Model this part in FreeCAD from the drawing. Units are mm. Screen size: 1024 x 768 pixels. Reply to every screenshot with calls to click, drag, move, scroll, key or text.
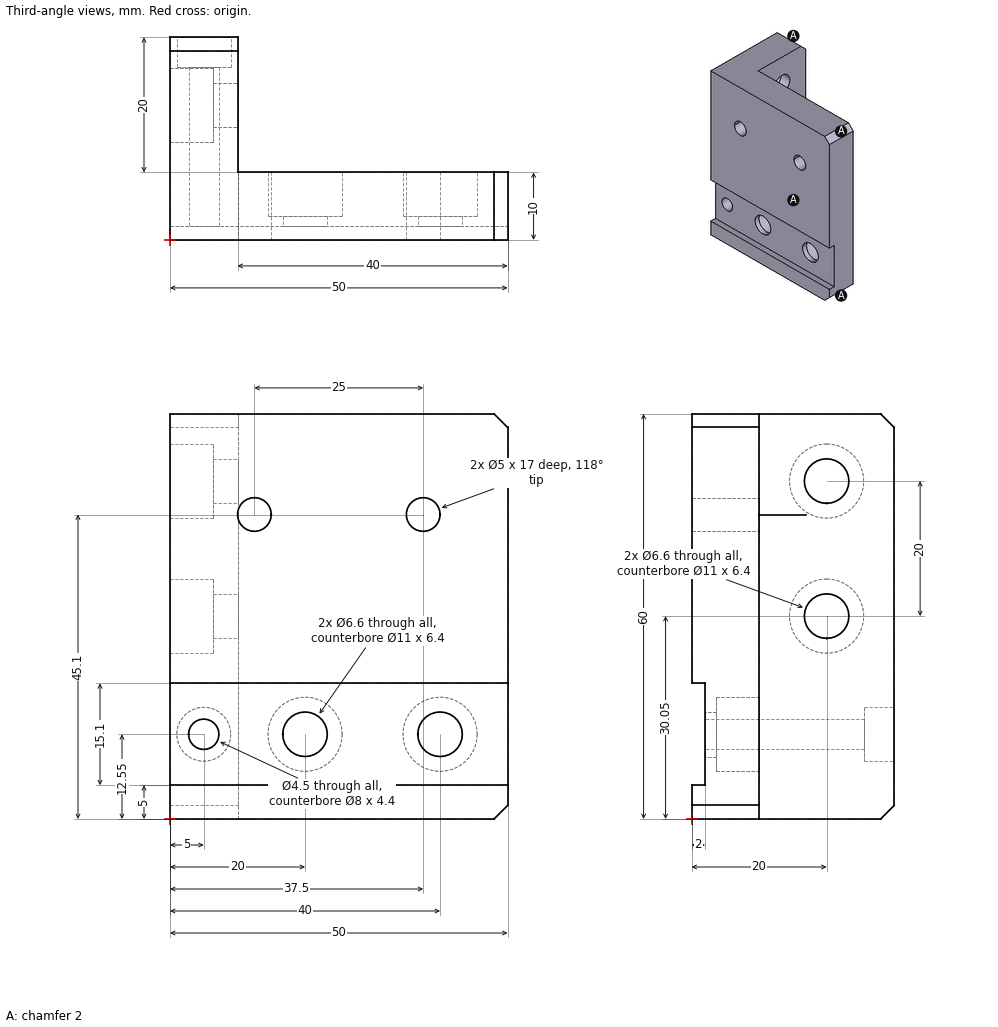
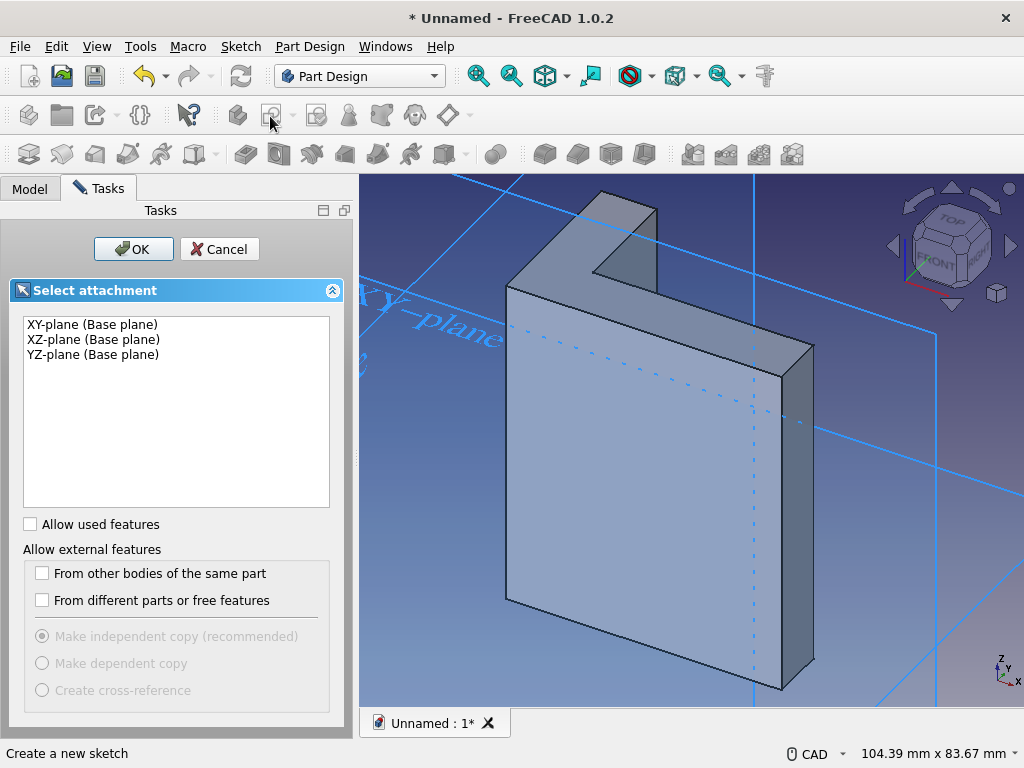
click(84, 340)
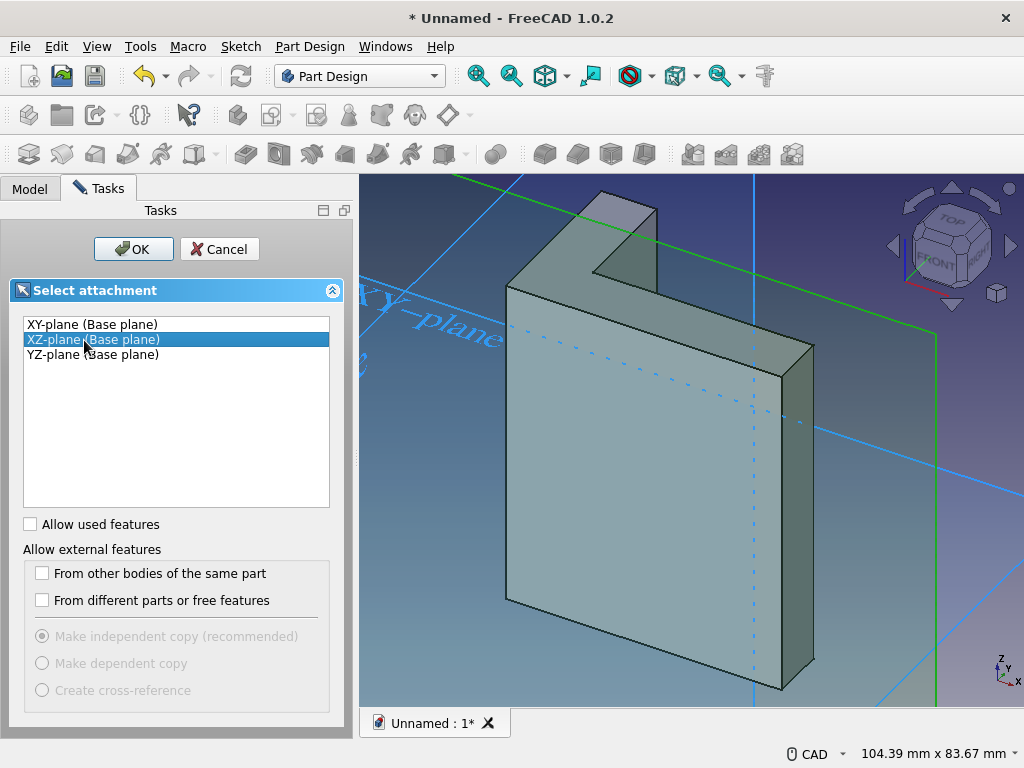
click(134, 249)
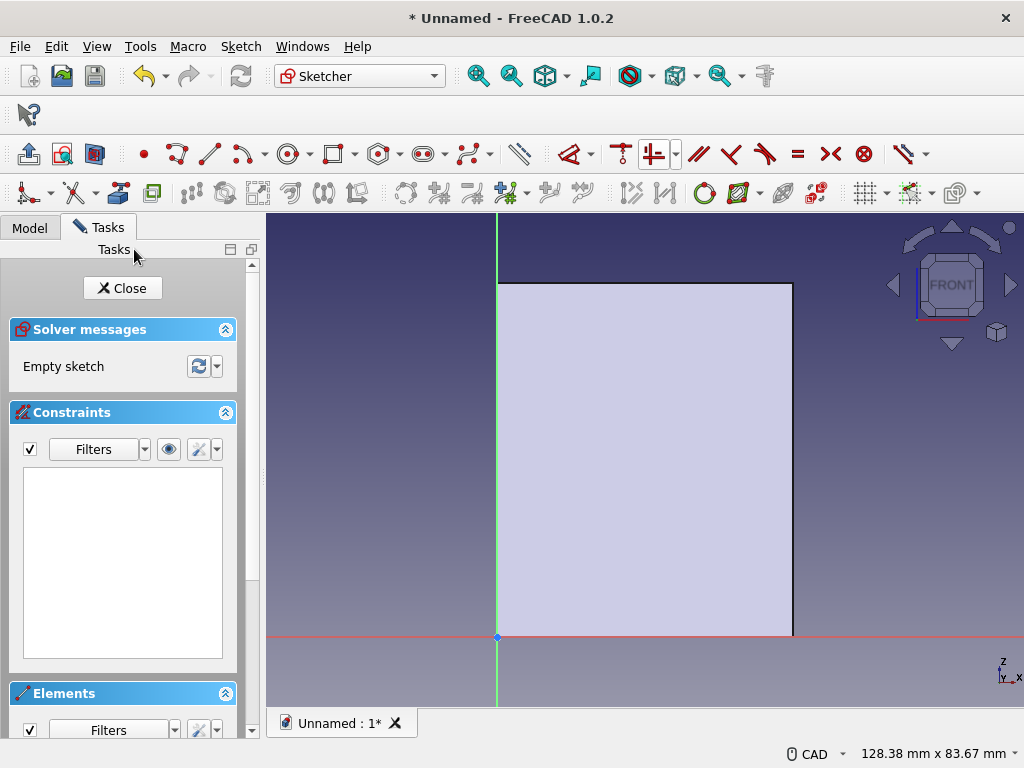
scroll(784, 679, up, 2)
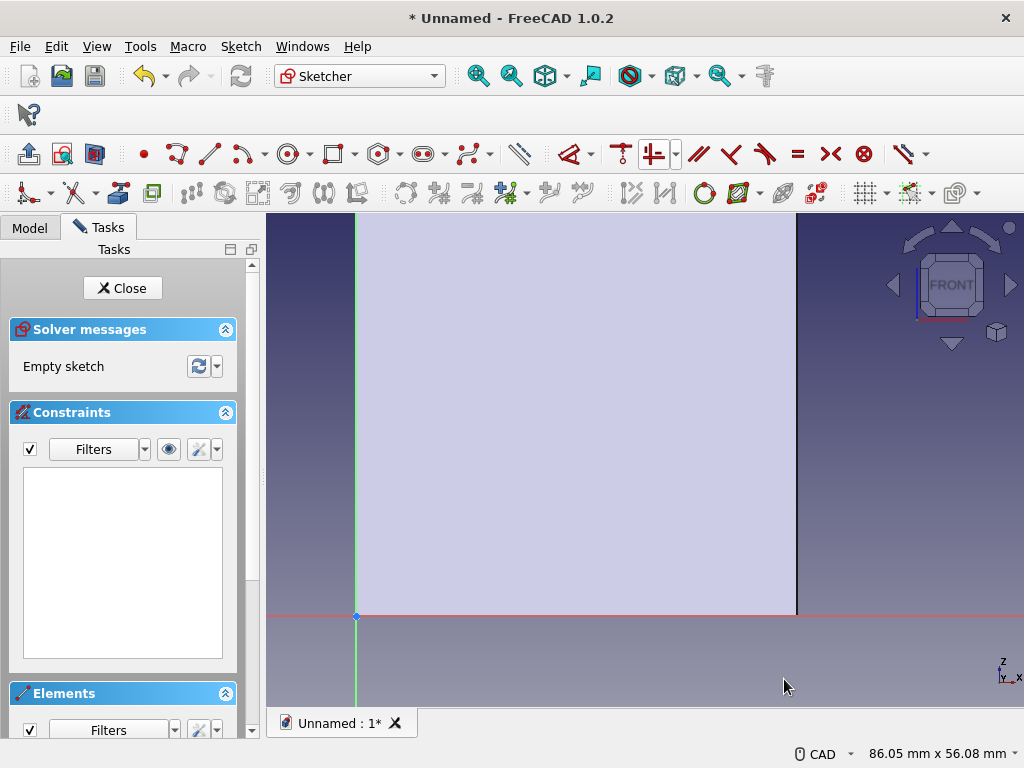
click(332, 154)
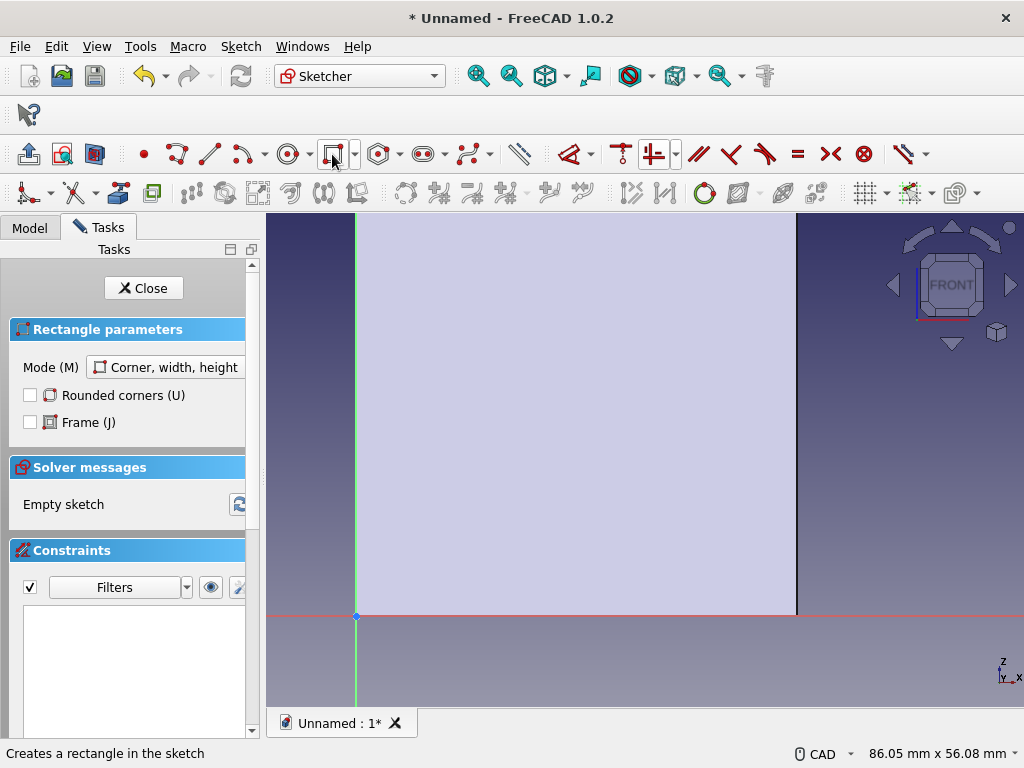
click(356, 439)
click(797, 572)
key(Escape)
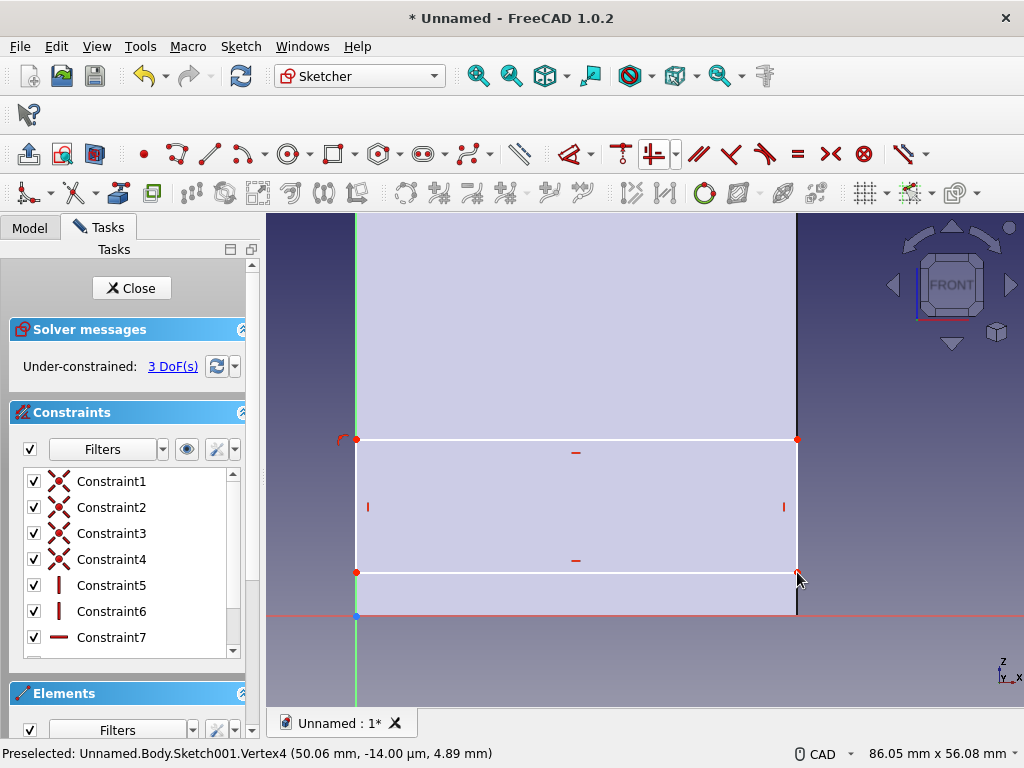
click(568, 154)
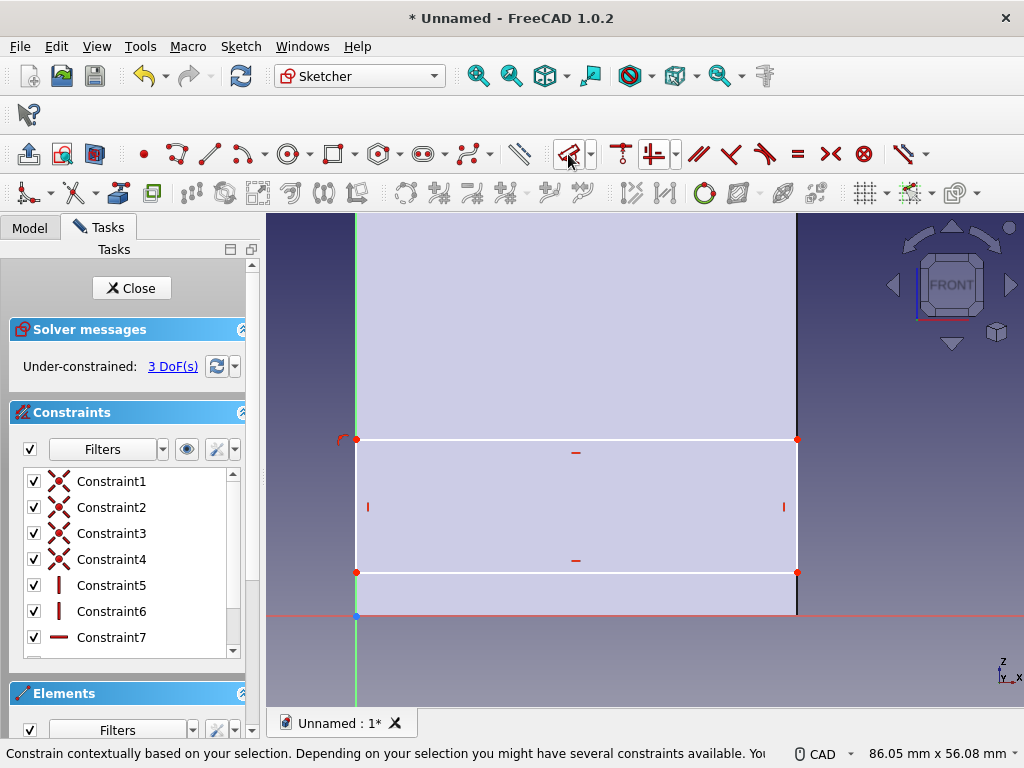
click(488, 573)
click(577, 539)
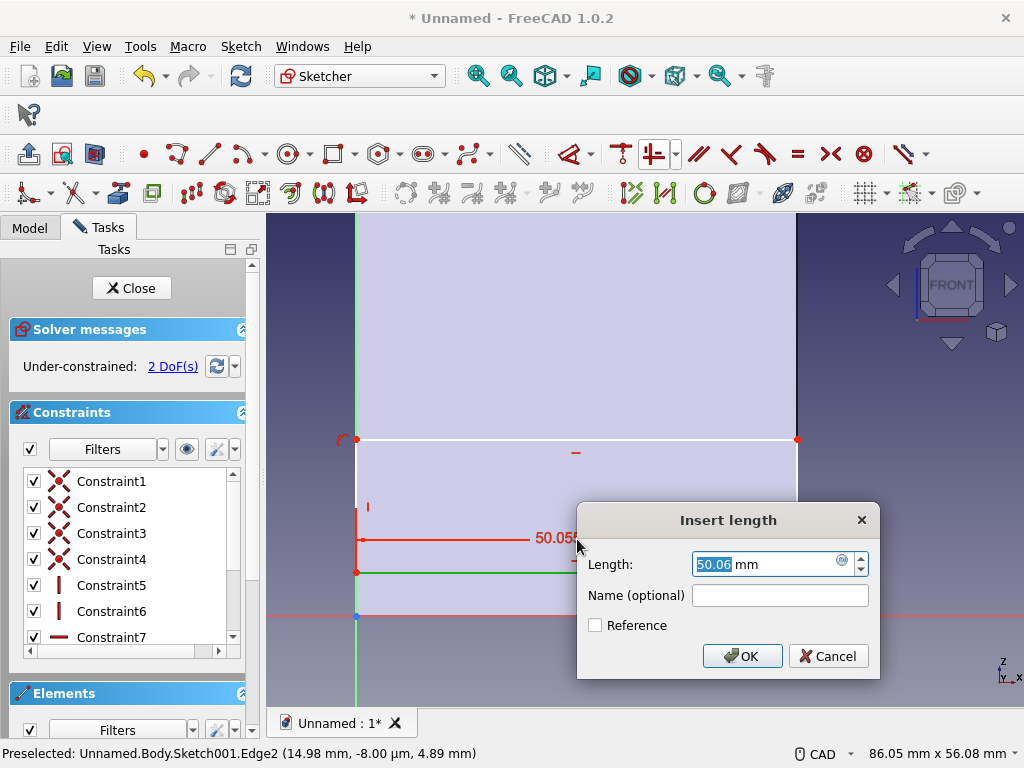
text(50)
key(Return)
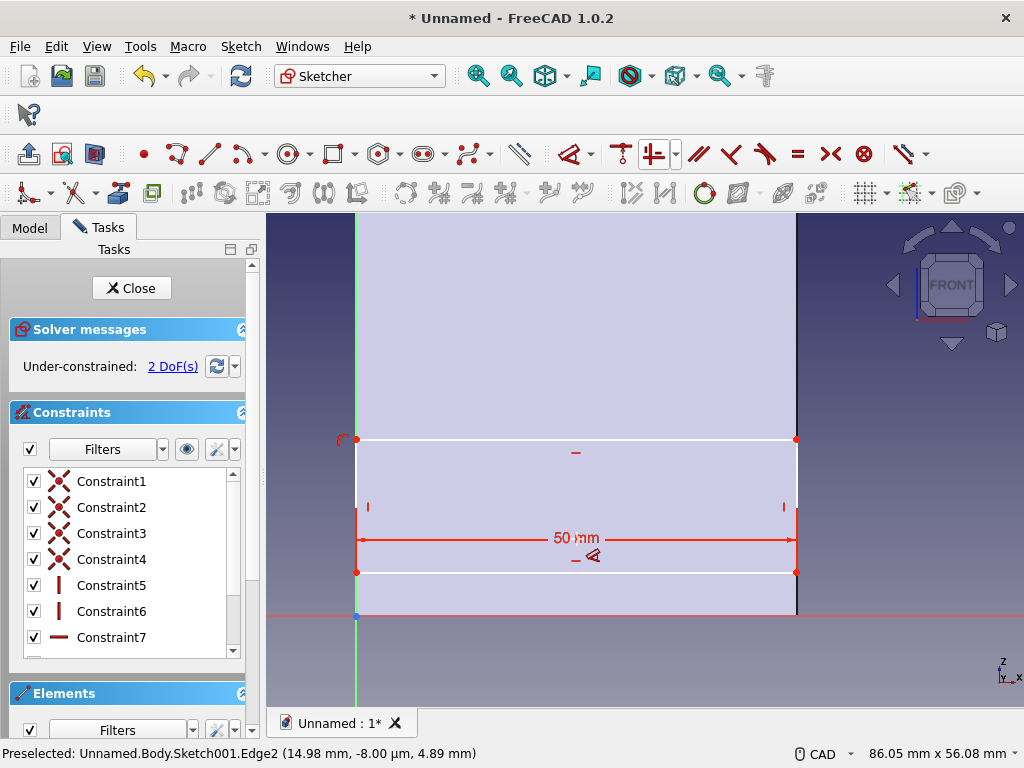
click(356, 573)
click(322, 595)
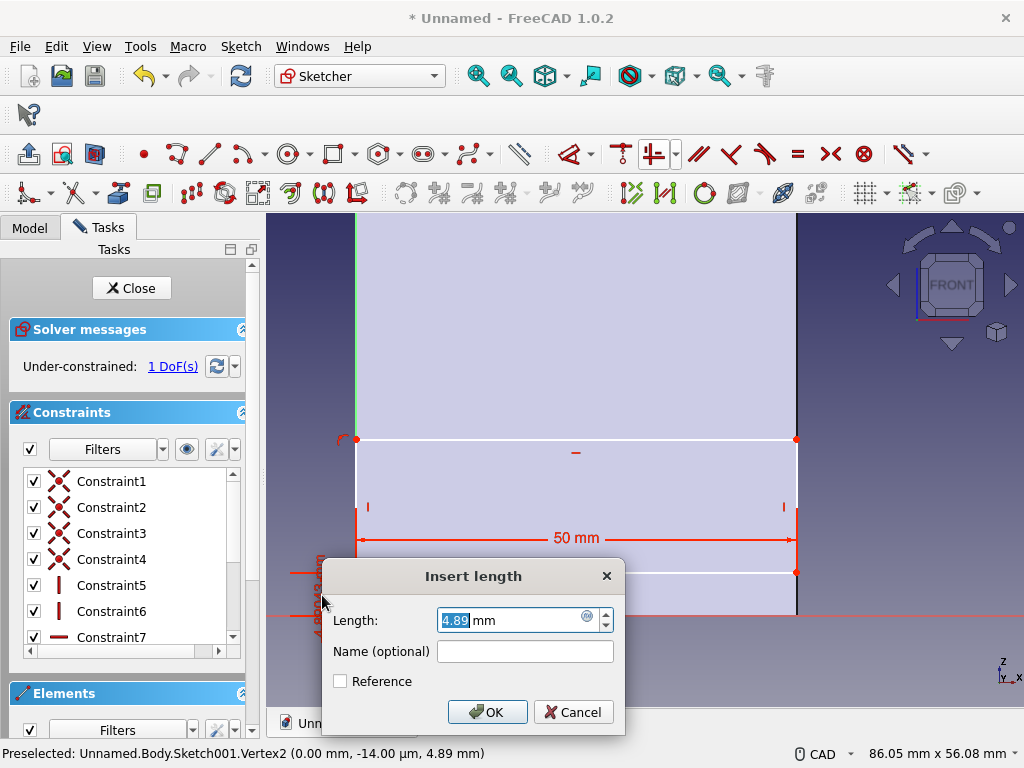
text(5)
key(Return)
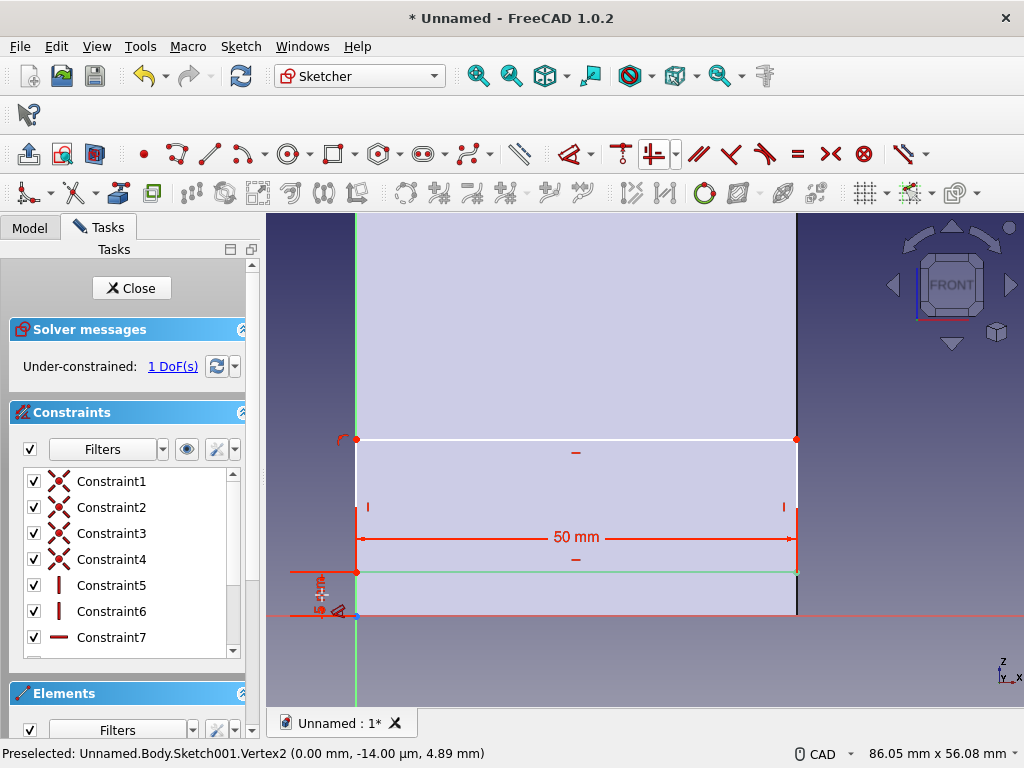
click(356, 480)
click(322, 506)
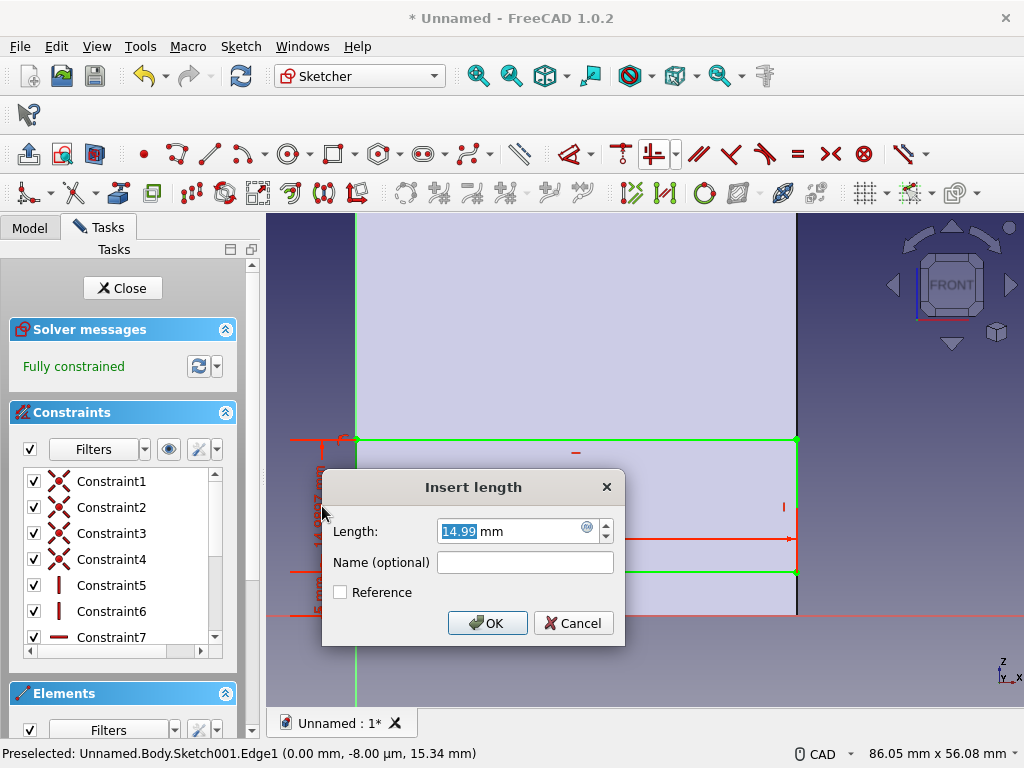
text(15.1)
key(Return)
key(Escape)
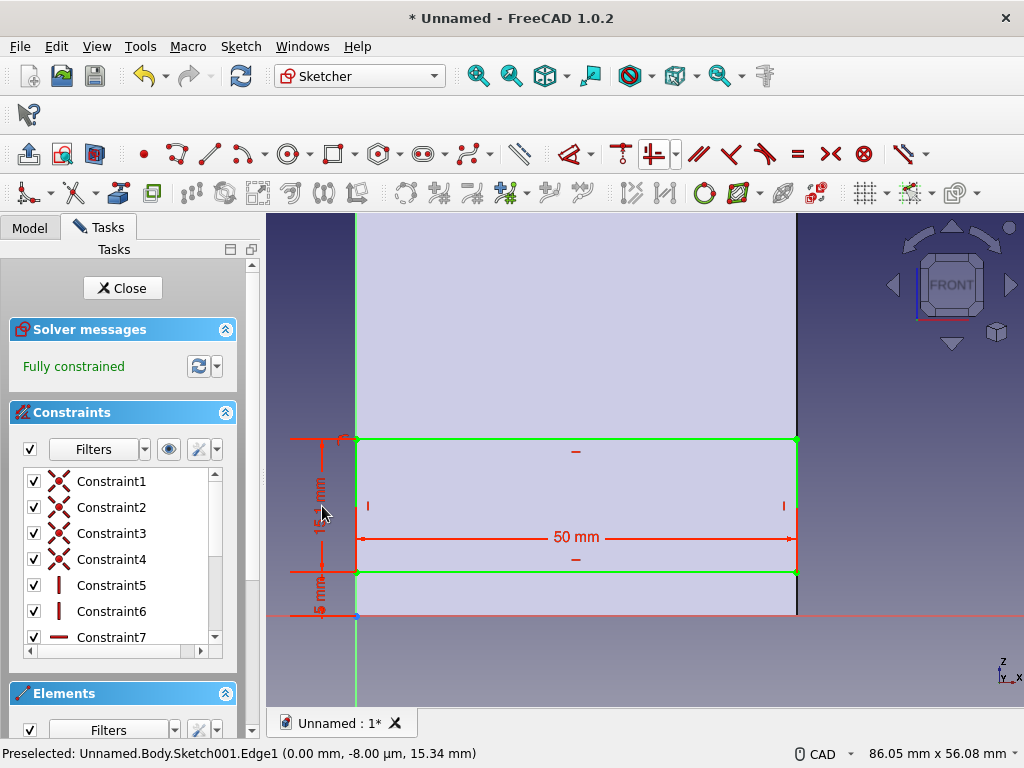
click(123, 288)